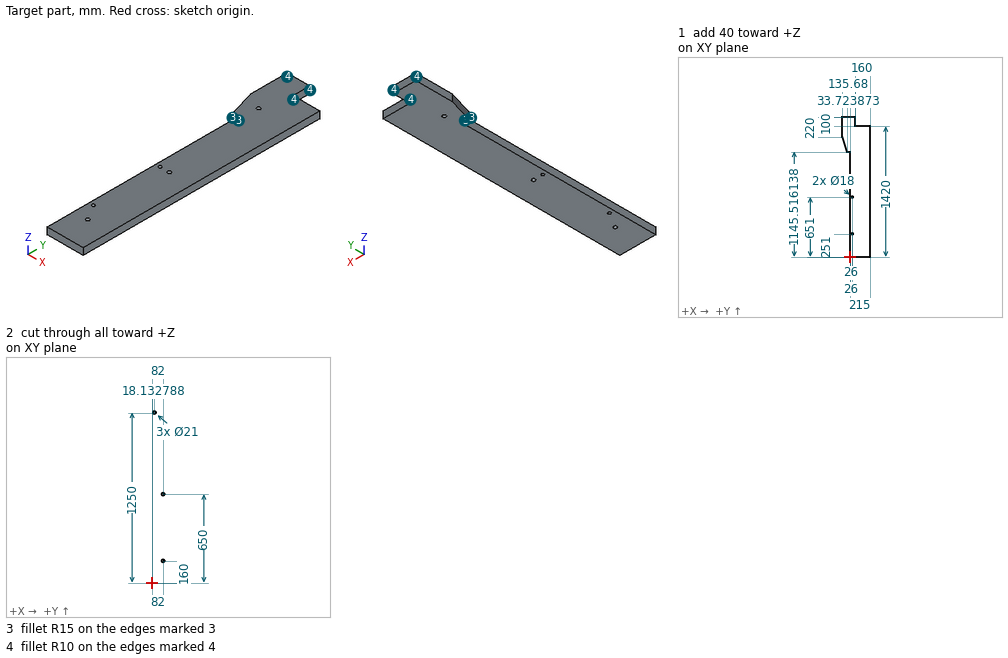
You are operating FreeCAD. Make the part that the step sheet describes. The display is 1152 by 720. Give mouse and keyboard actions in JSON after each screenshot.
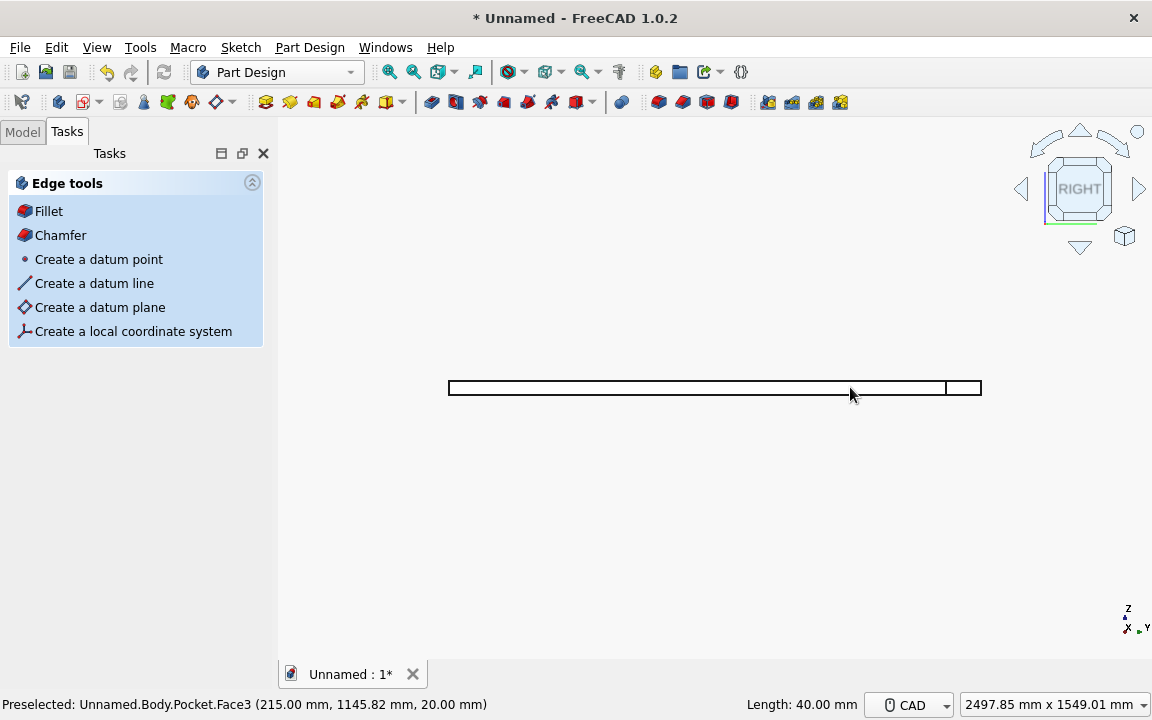
{"action": "key", "text": "5"}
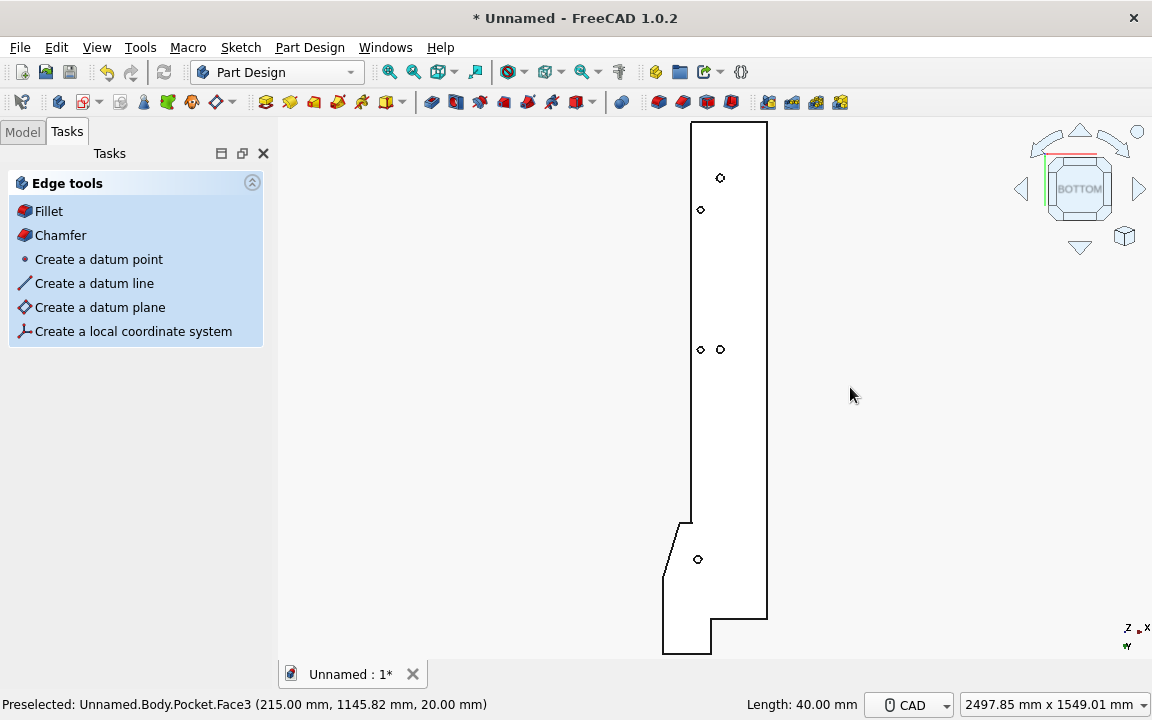
{"action": "scroll", "coordinate": [692, 522], "scroll_direction": "up", "scroll_amount": 6}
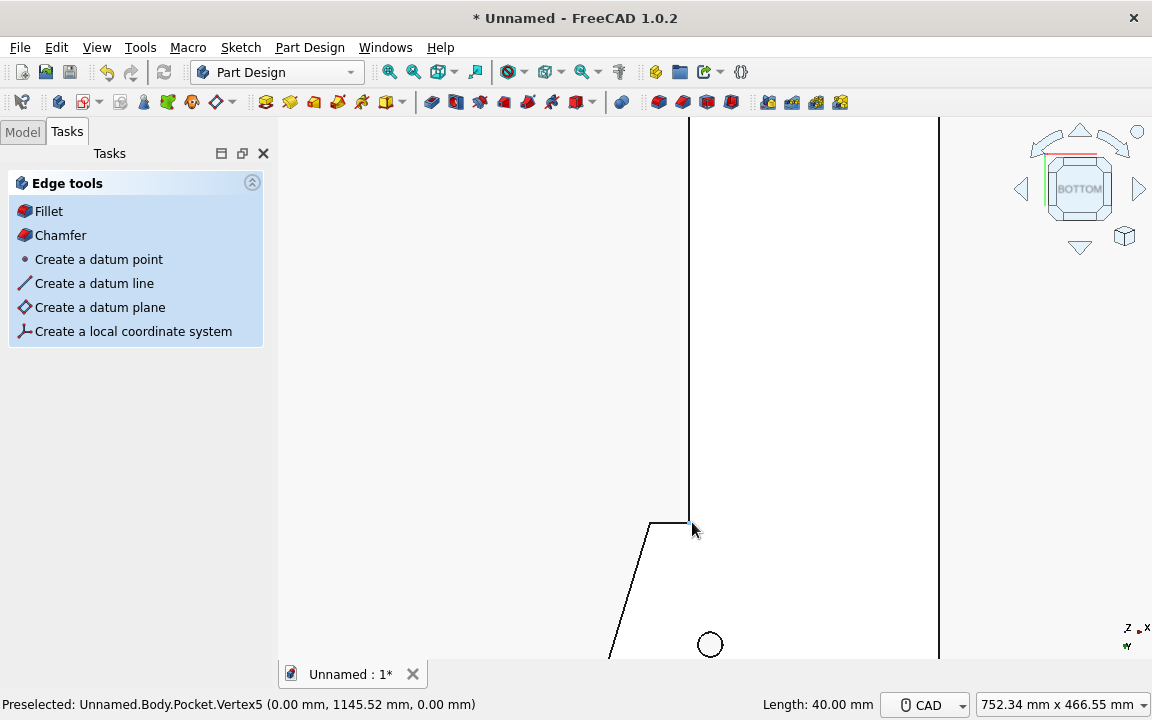
{"action": "left_click", "coordinate": [390, 72]}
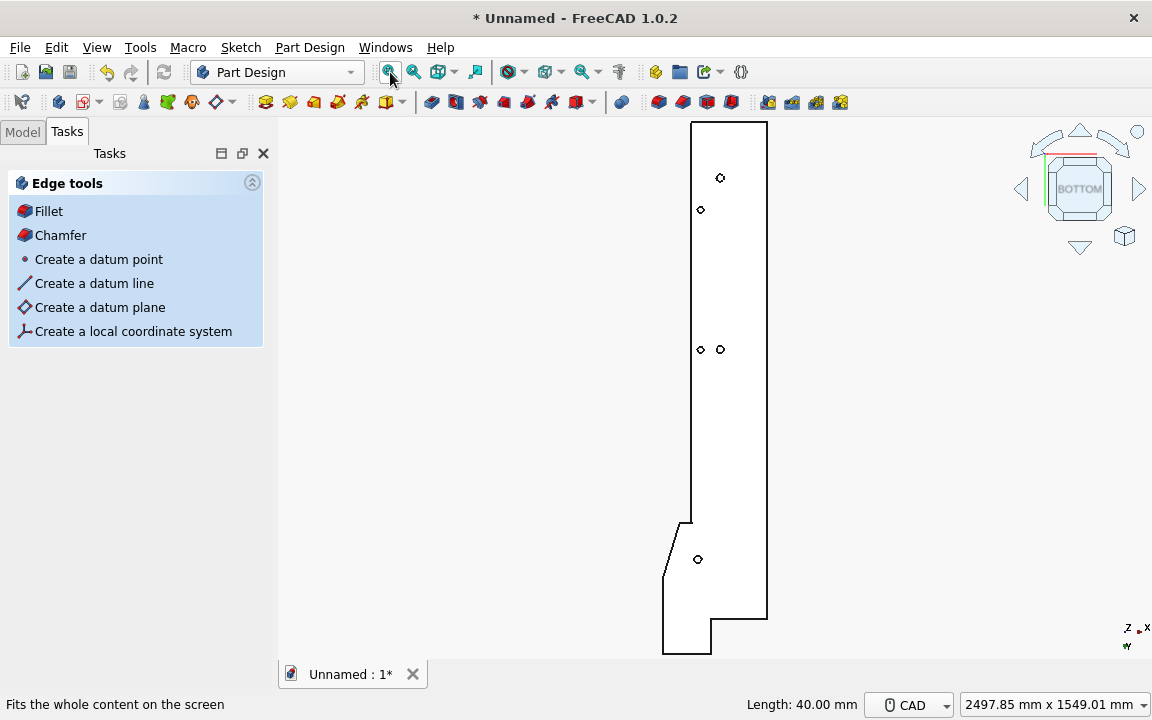
{"action": "key", "text": "4"}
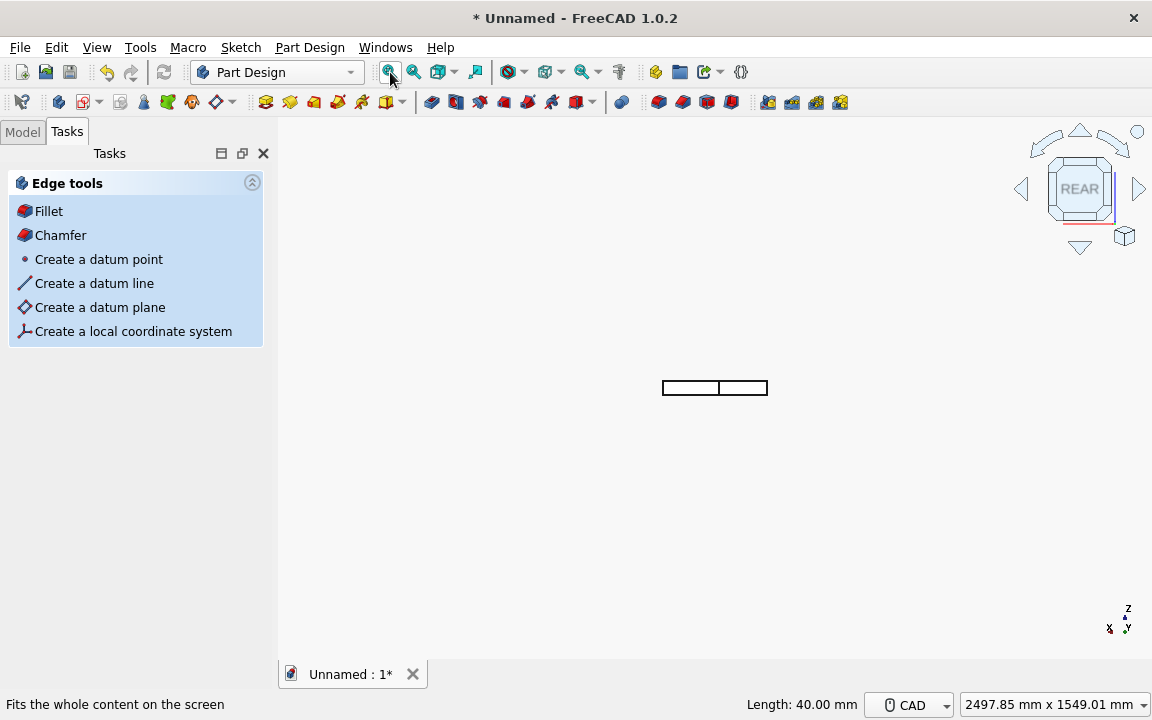
{"action": "key", "text": "v f"}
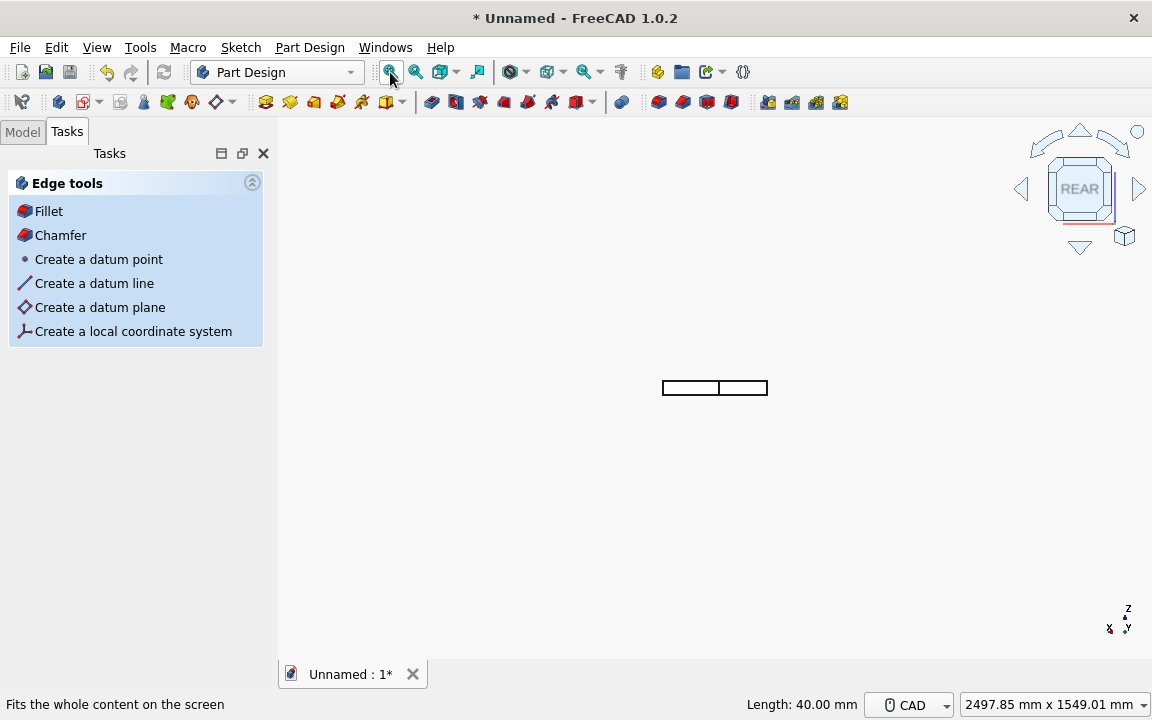
{"action": "scroll", "coordinate": [738, 387], "scroll_direction": "up", "scroll_amount": 6}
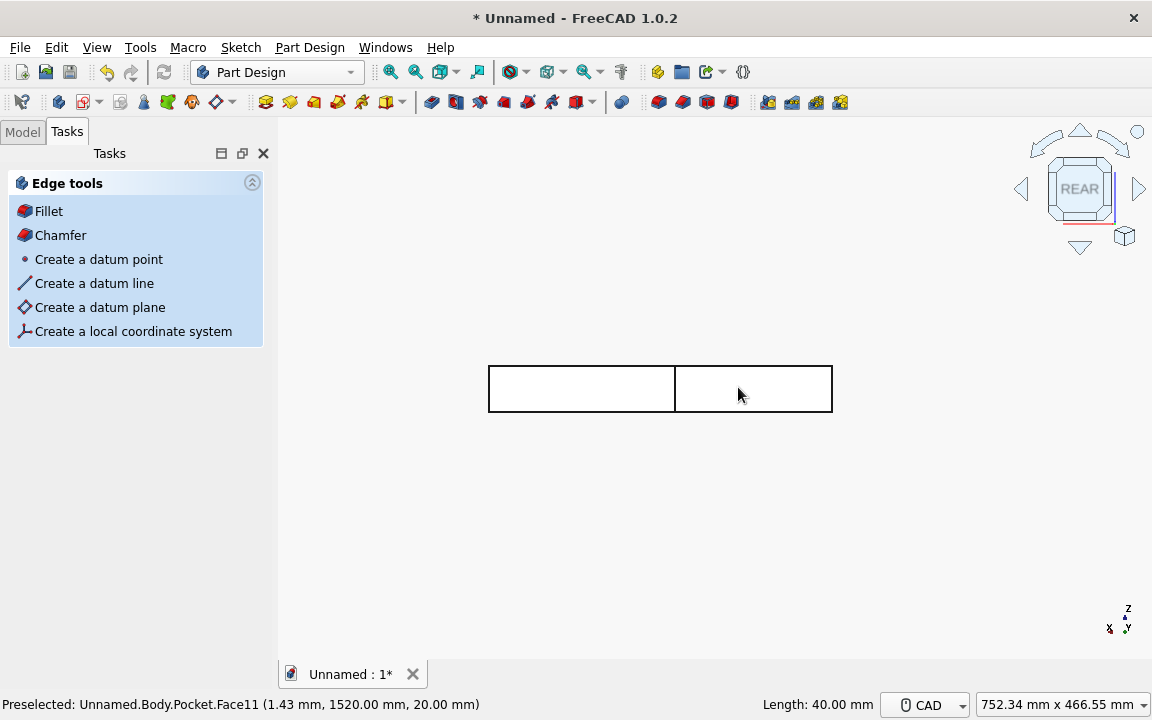
{"action": "left_click", "coordinate": [392, 72]}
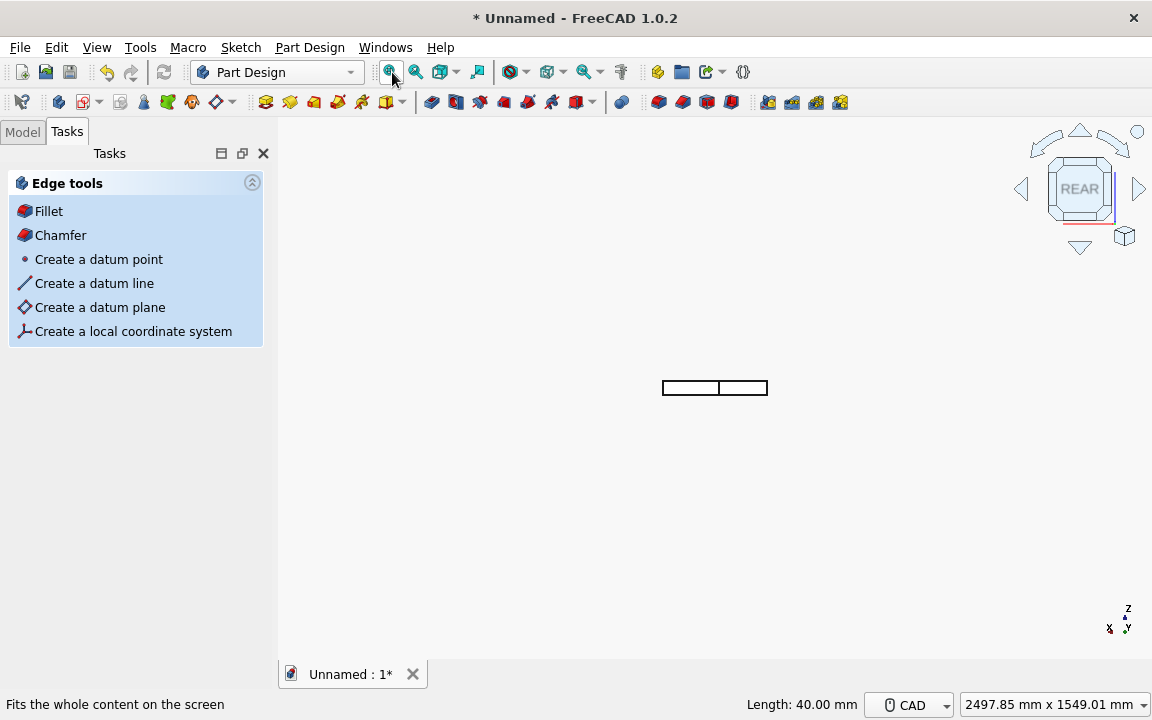
{"action": "key", "text": "6"}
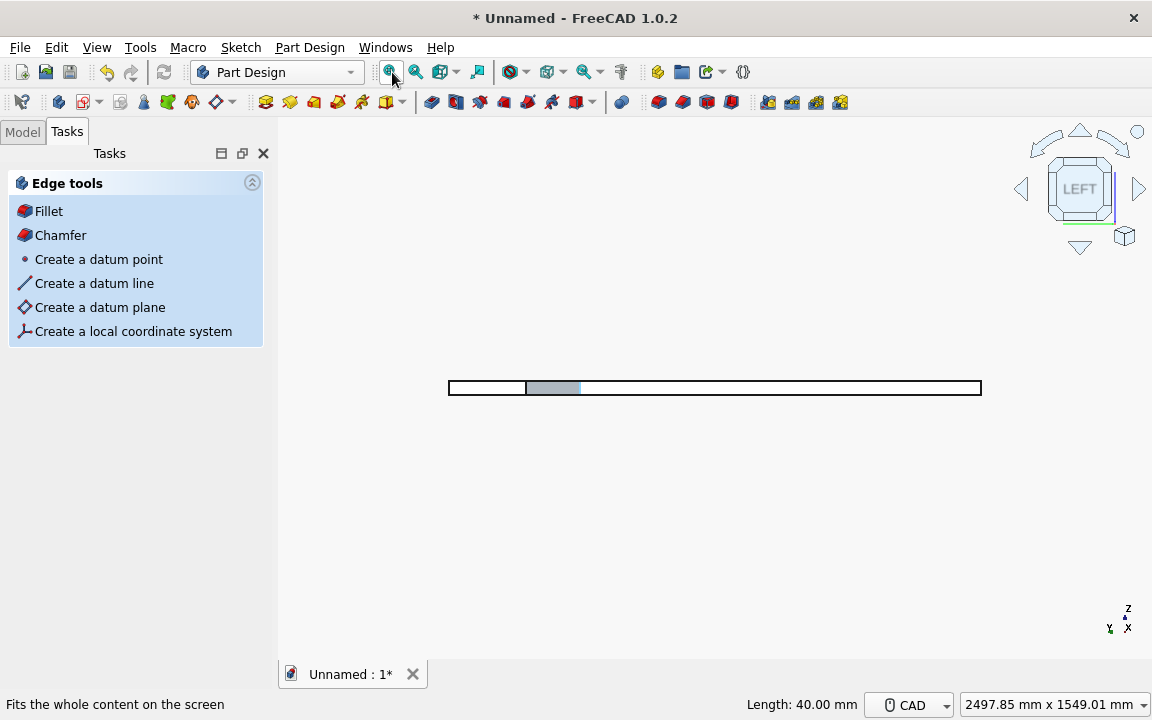
{"action": "scroll", "coordinate": [580, 387], "scroll_direction": "up", "scroll_amount": 6}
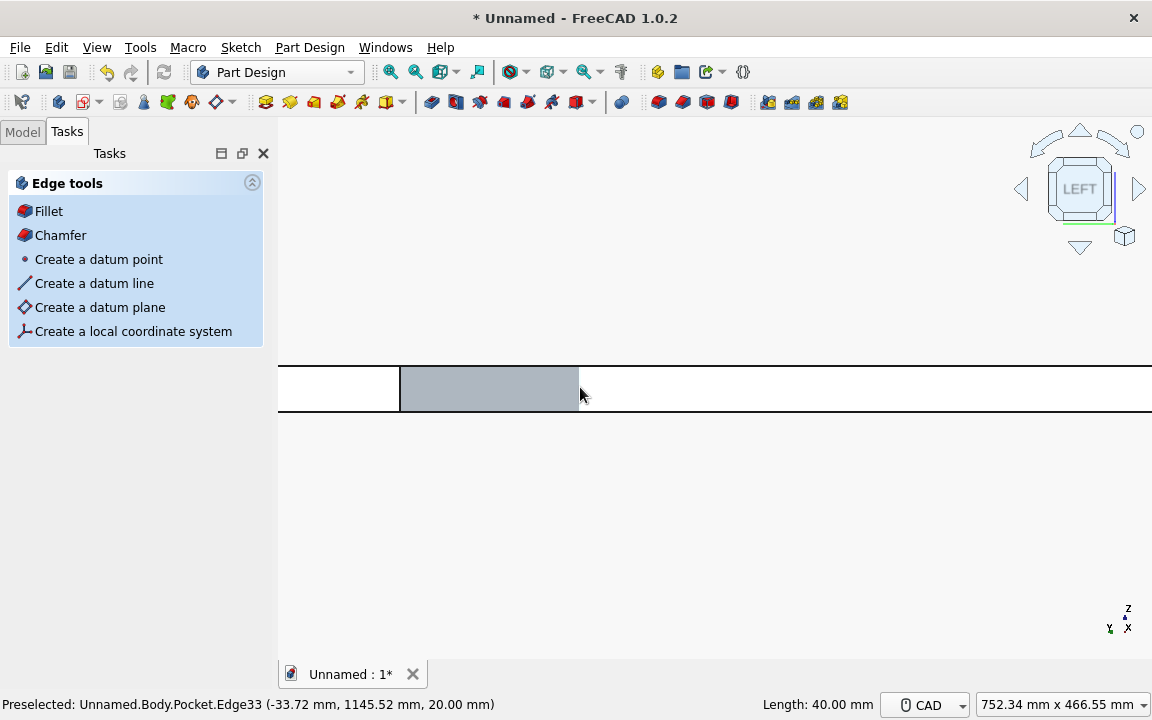
{"action": "key", "text": "v f"}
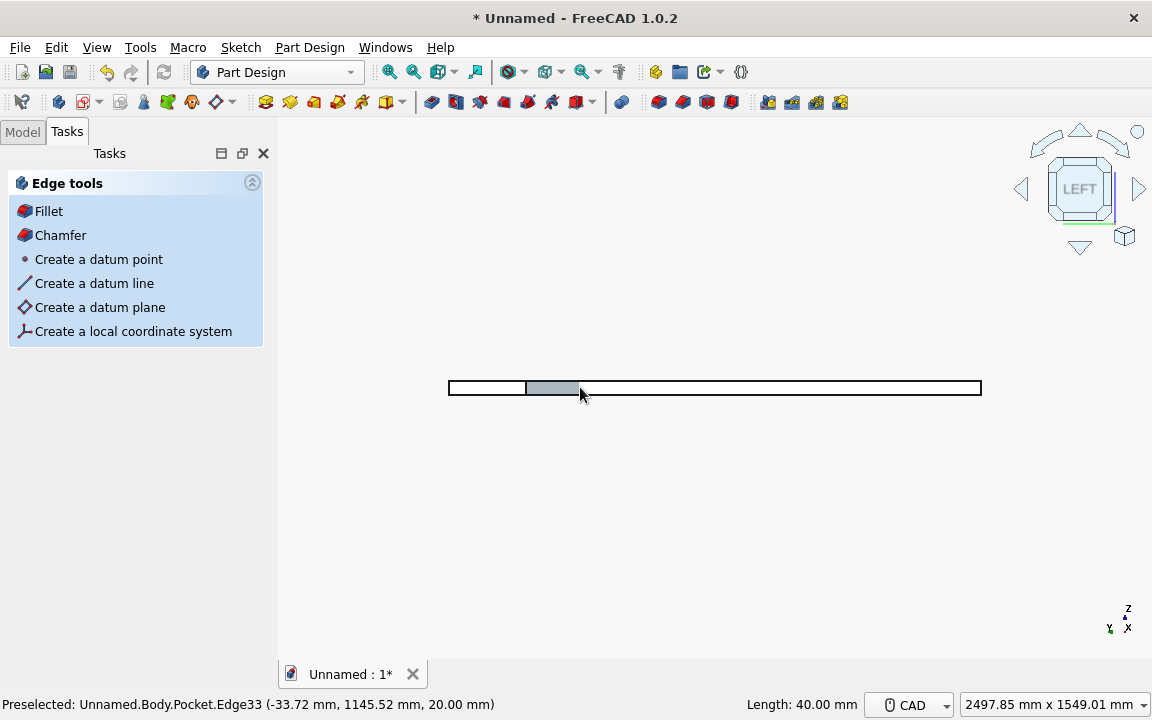
{"action": "key", "text": "v 3"}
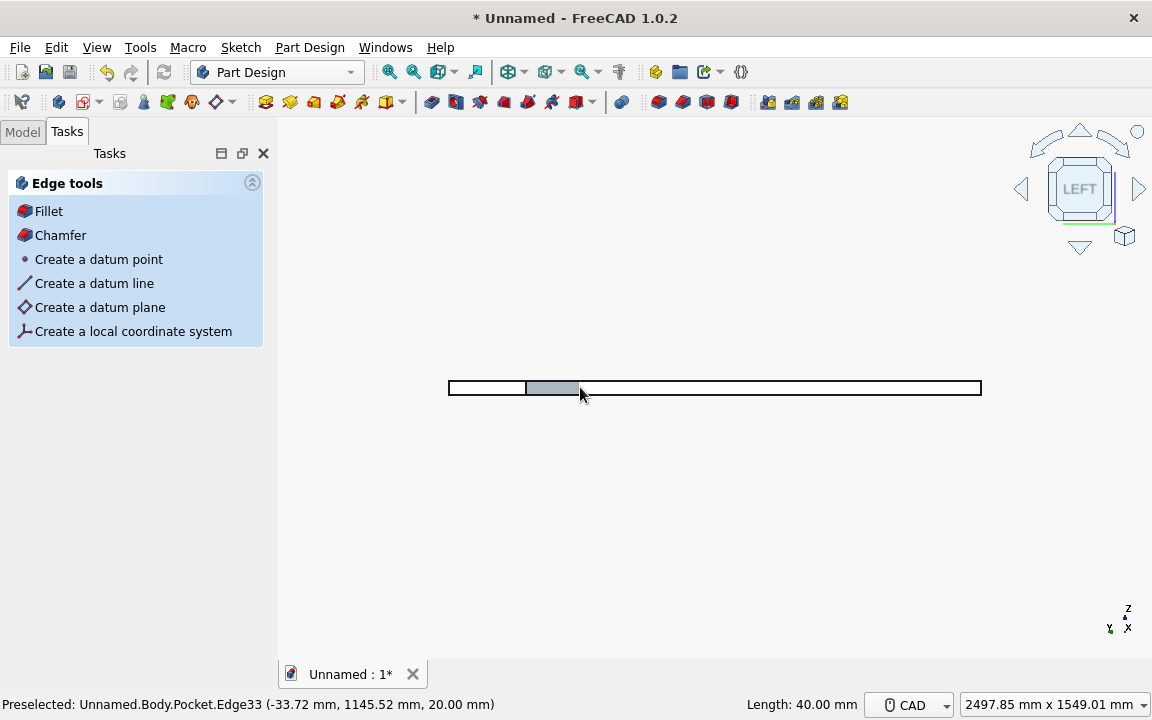
{"action": "key", "text": "0"}